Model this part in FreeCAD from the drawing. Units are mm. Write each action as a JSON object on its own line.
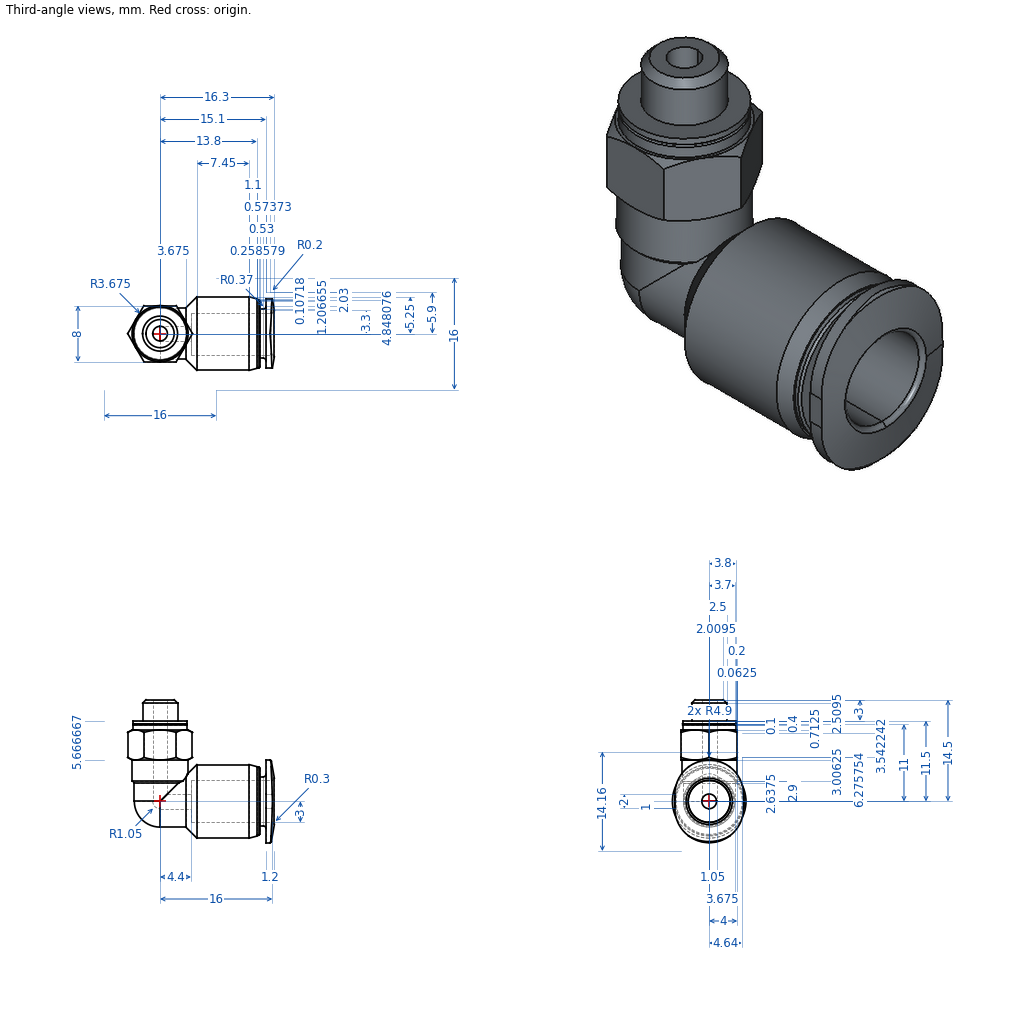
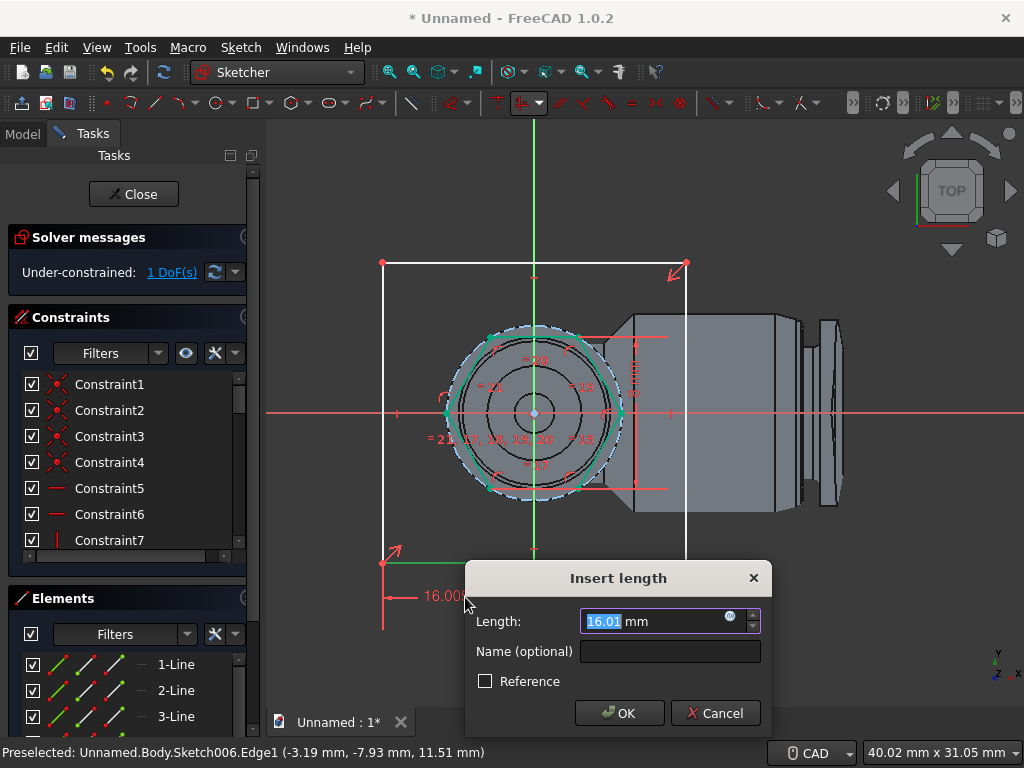
{"action": "type", "text": "16"}
{"action": "key", "text": "Return"}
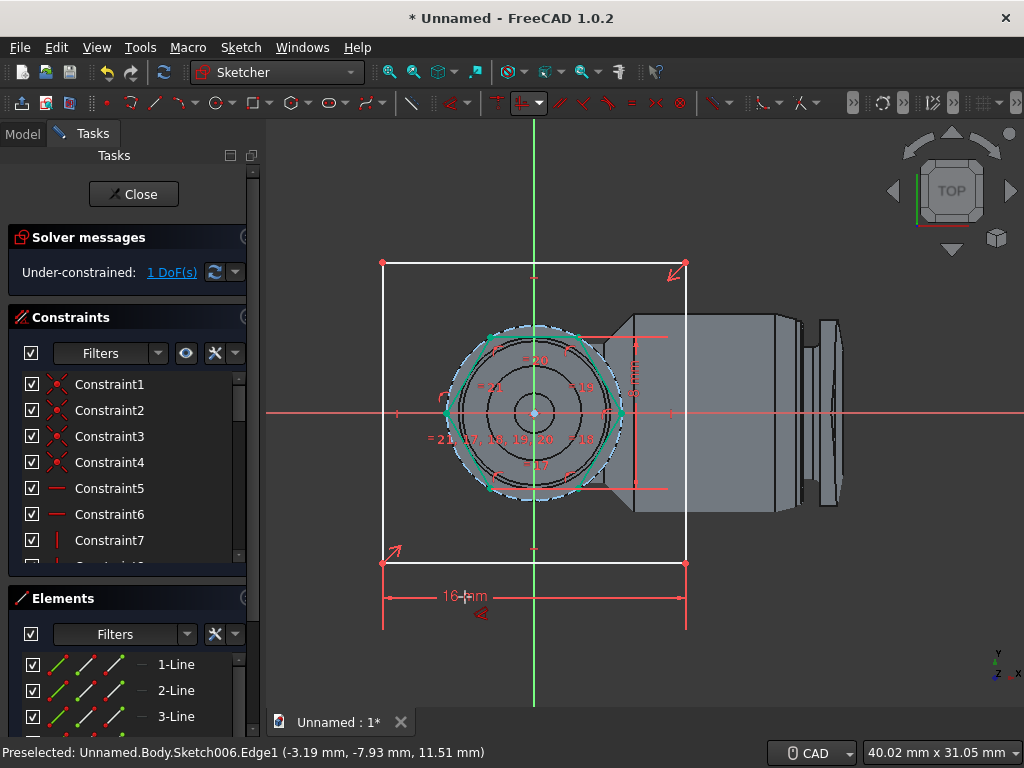
{"action": "left_click", "coordinate": [686, 473]}
{"action": "left_click", "coordinate": [720, 344]}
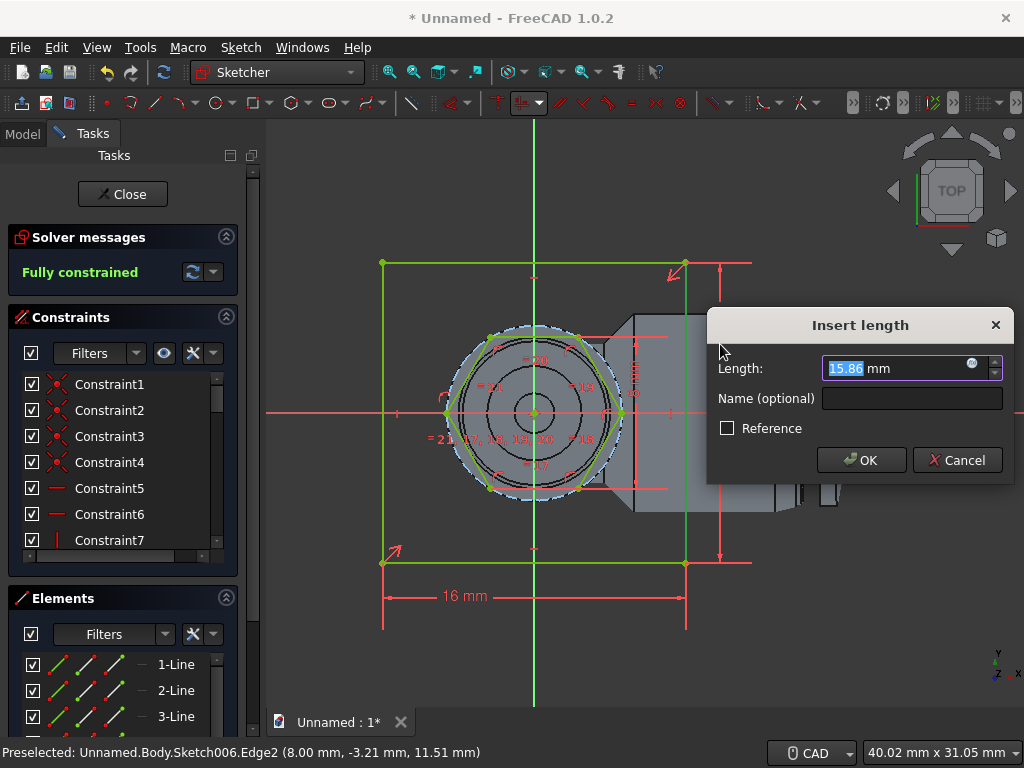
{"action": "type", "text": "16"}
{"action": "key", "text": "Return"}
{"action": "key", "text": "Escape"}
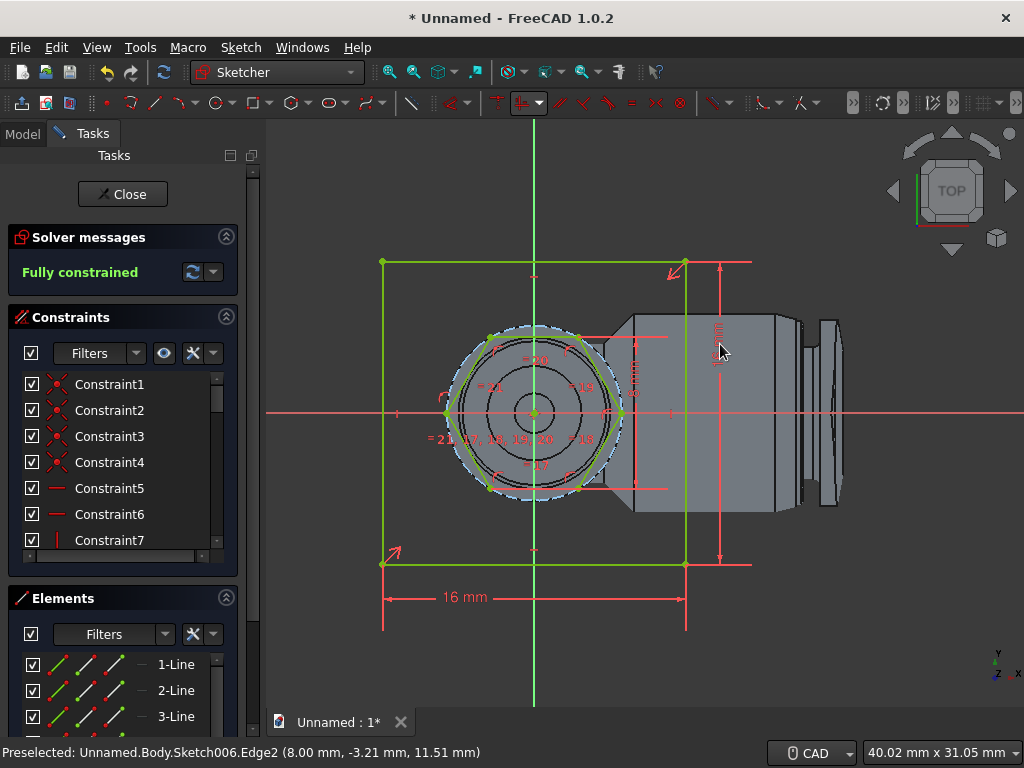
{"action": "left_click", "coordinate": [123, 194]}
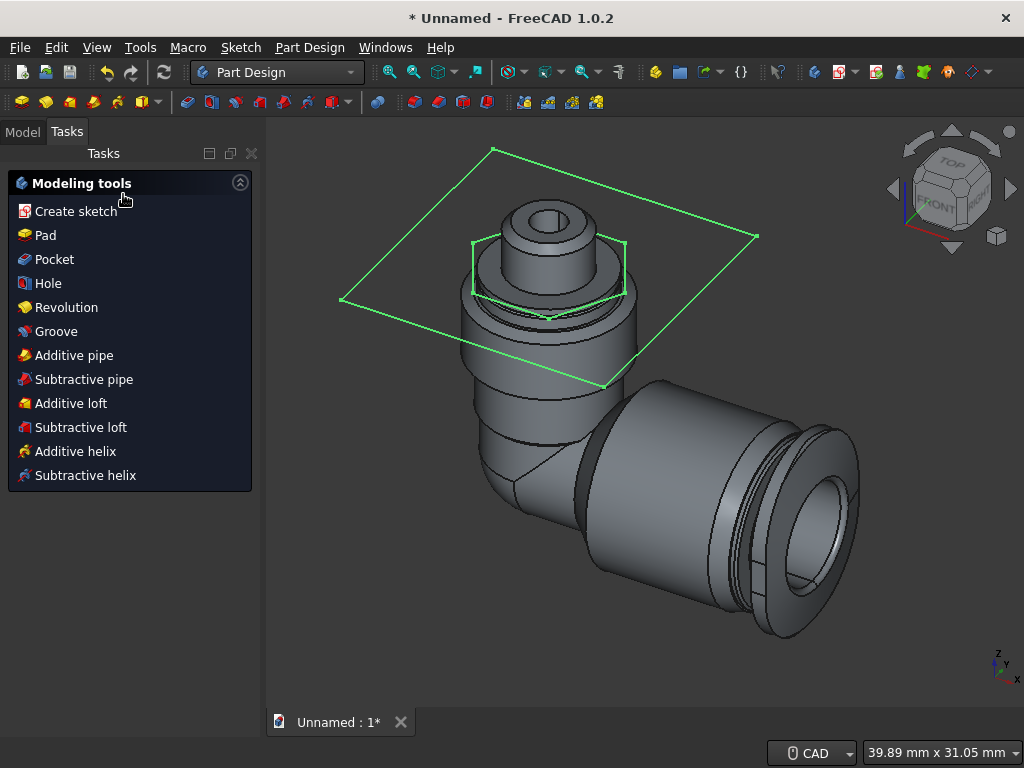
{"action": "left_click", "coordinate": [188, 102]}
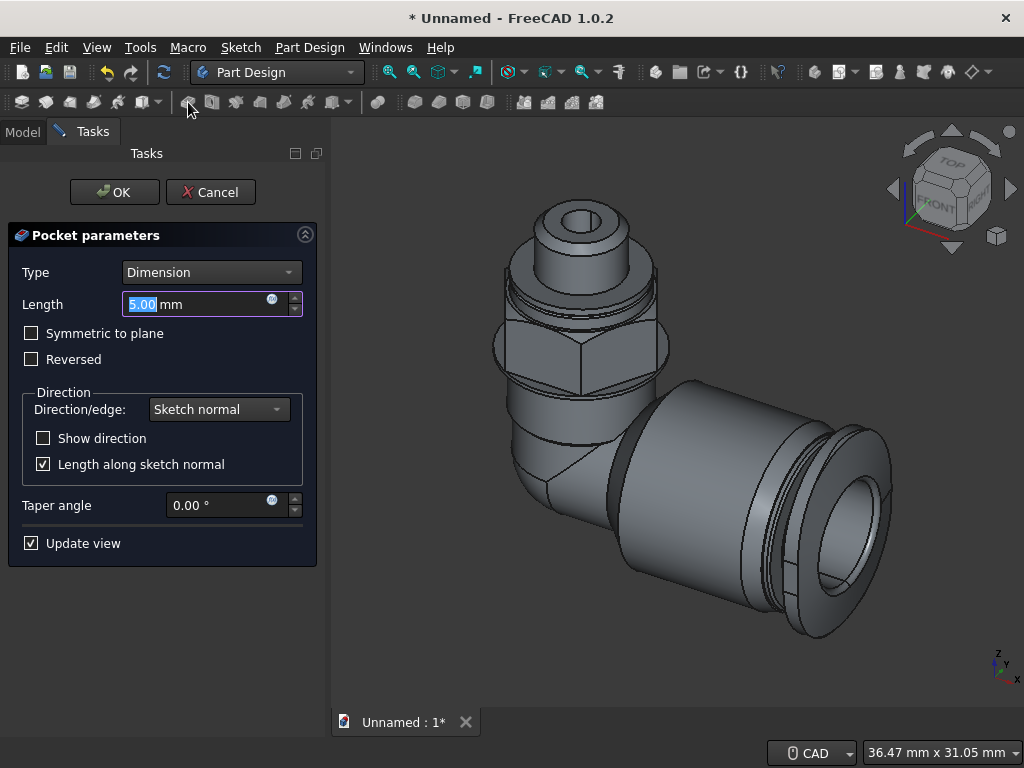
{"action": "type", "text": "5.666667"}
{"action": "key", "text": "Tab"}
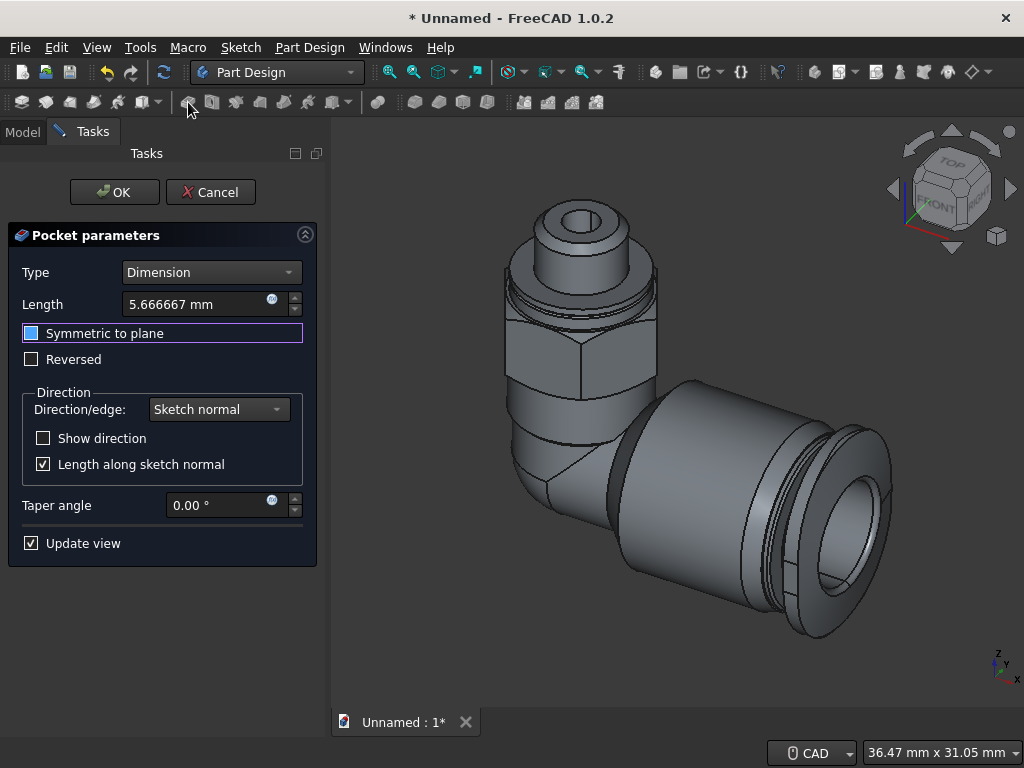
{"action": "left_click", "coordinate": [115, 192]}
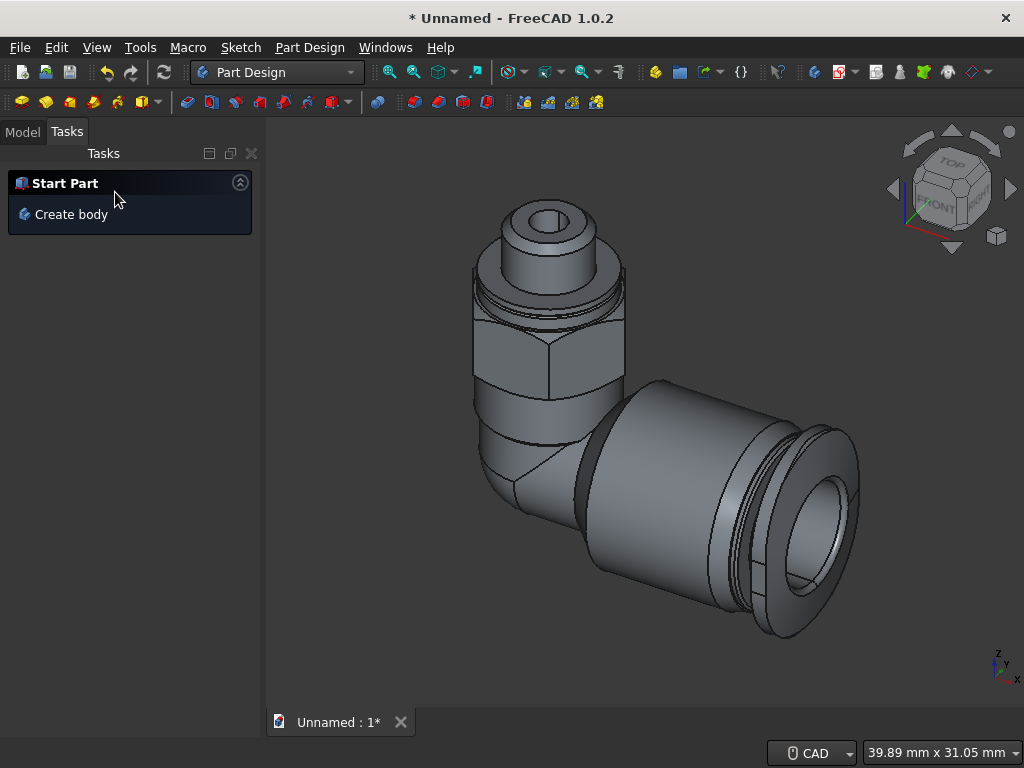
{"action": "key", "text": "0"}